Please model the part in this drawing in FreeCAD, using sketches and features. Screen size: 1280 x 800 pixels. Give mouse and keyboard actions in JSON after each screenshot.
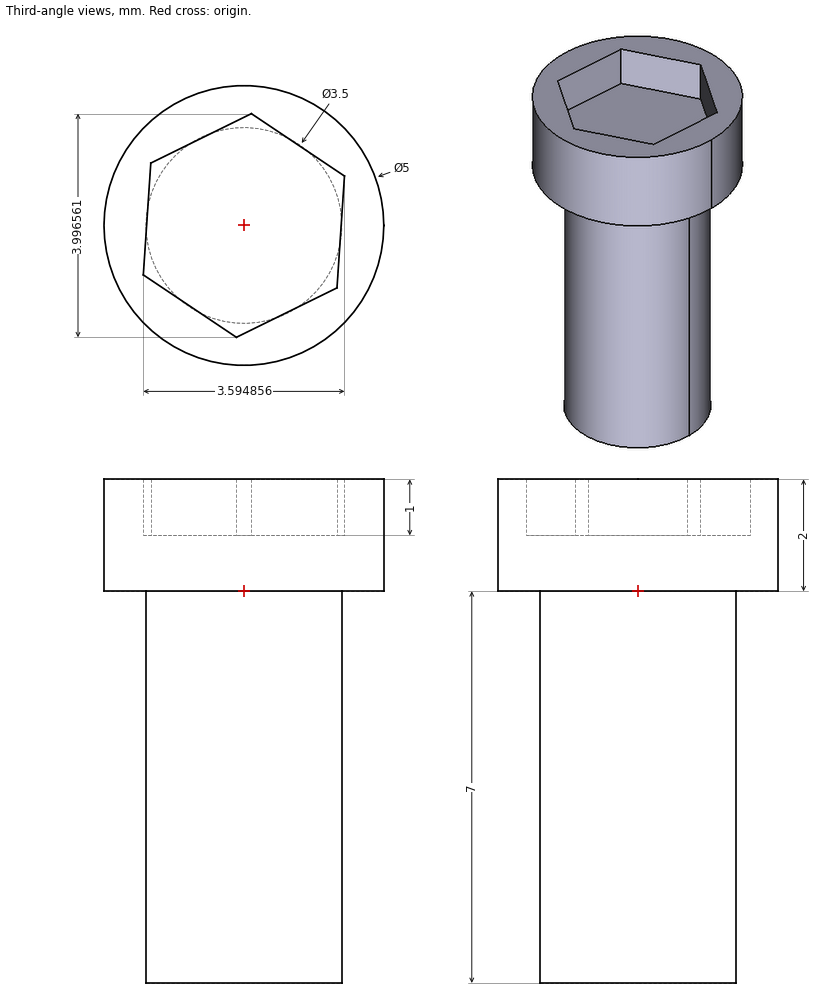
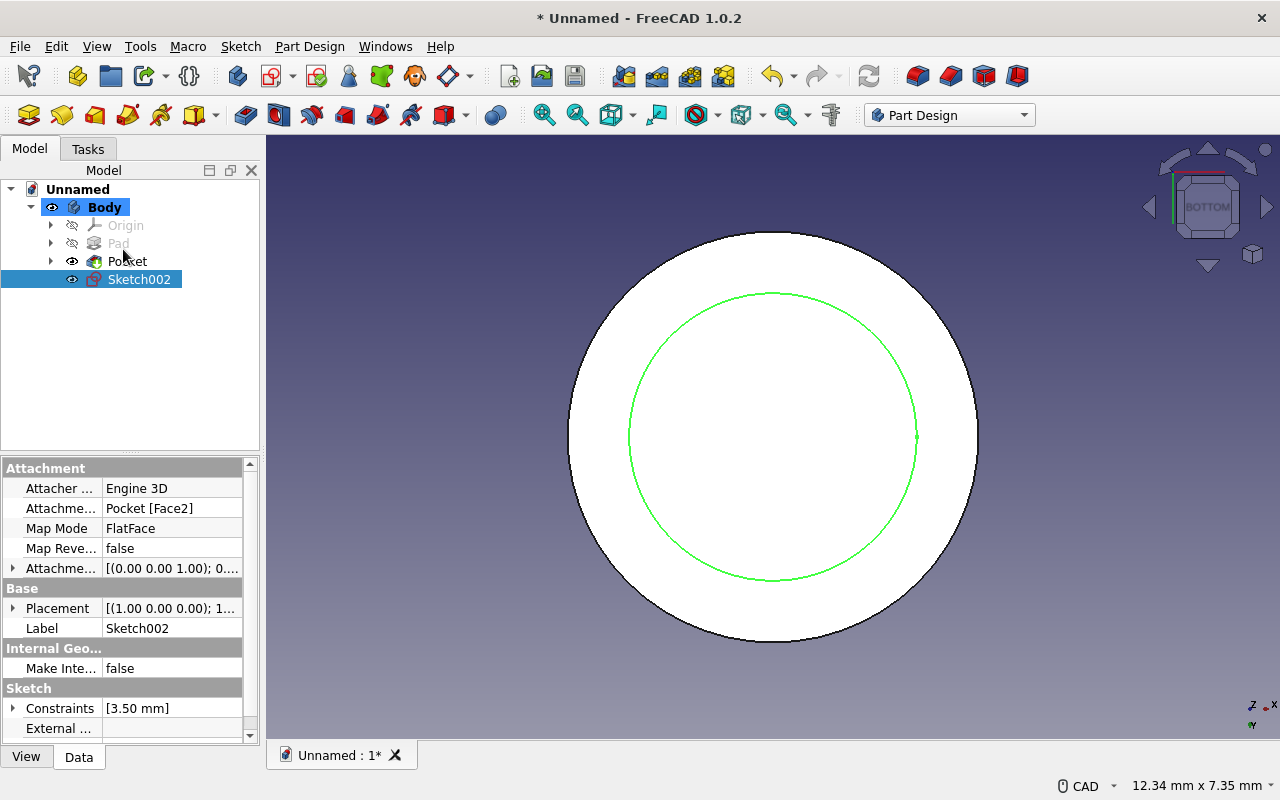
{"action": "left_click", "coordinate": [29, 116]}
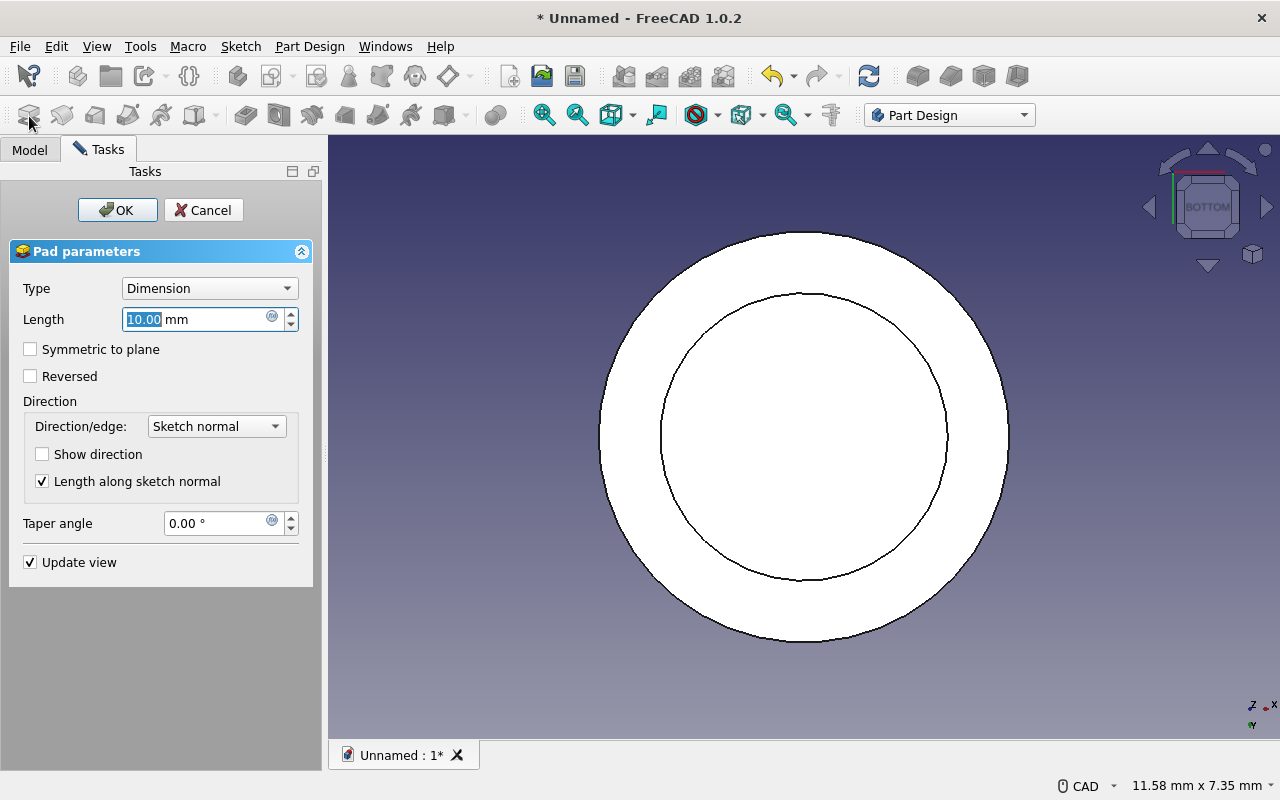
{"action": "type", "text": "7"}
{"action": "key", "text": "Tab"}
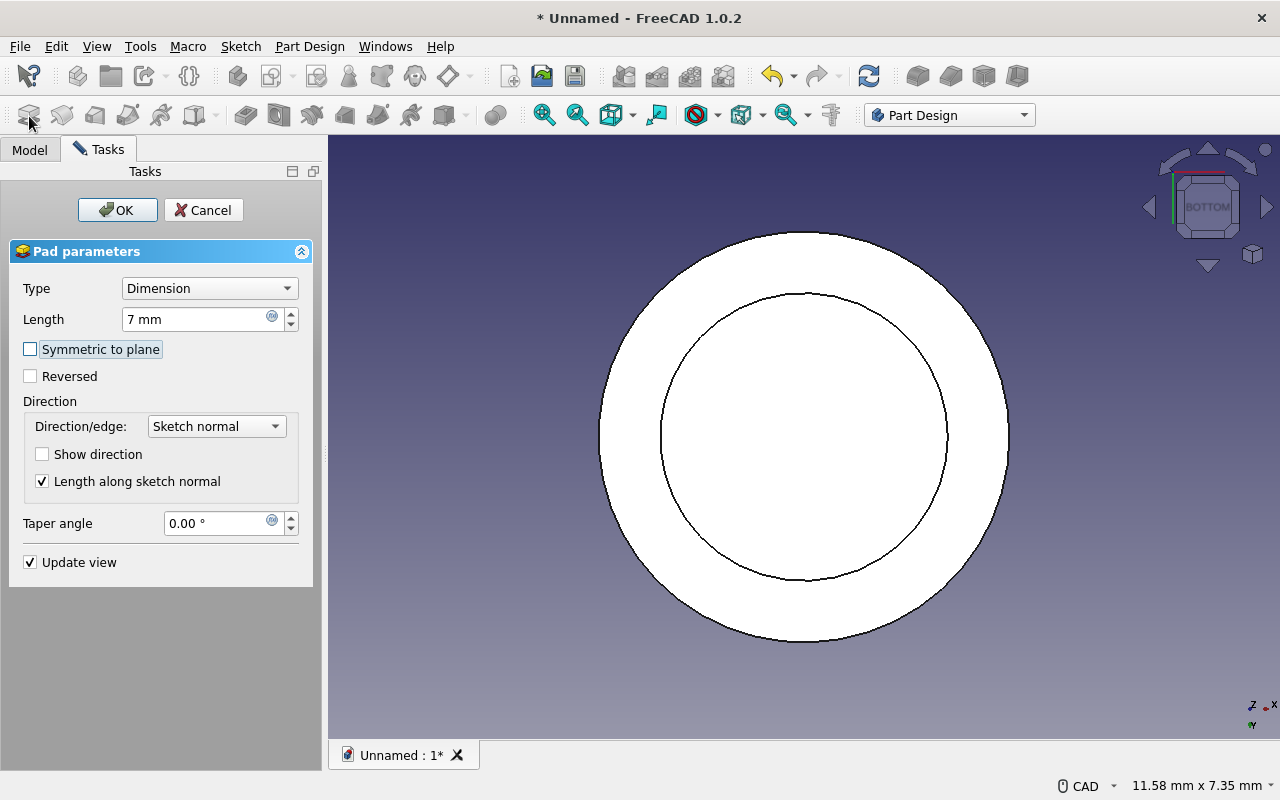
{"action": "left_click", "coordinate": [118, 210]}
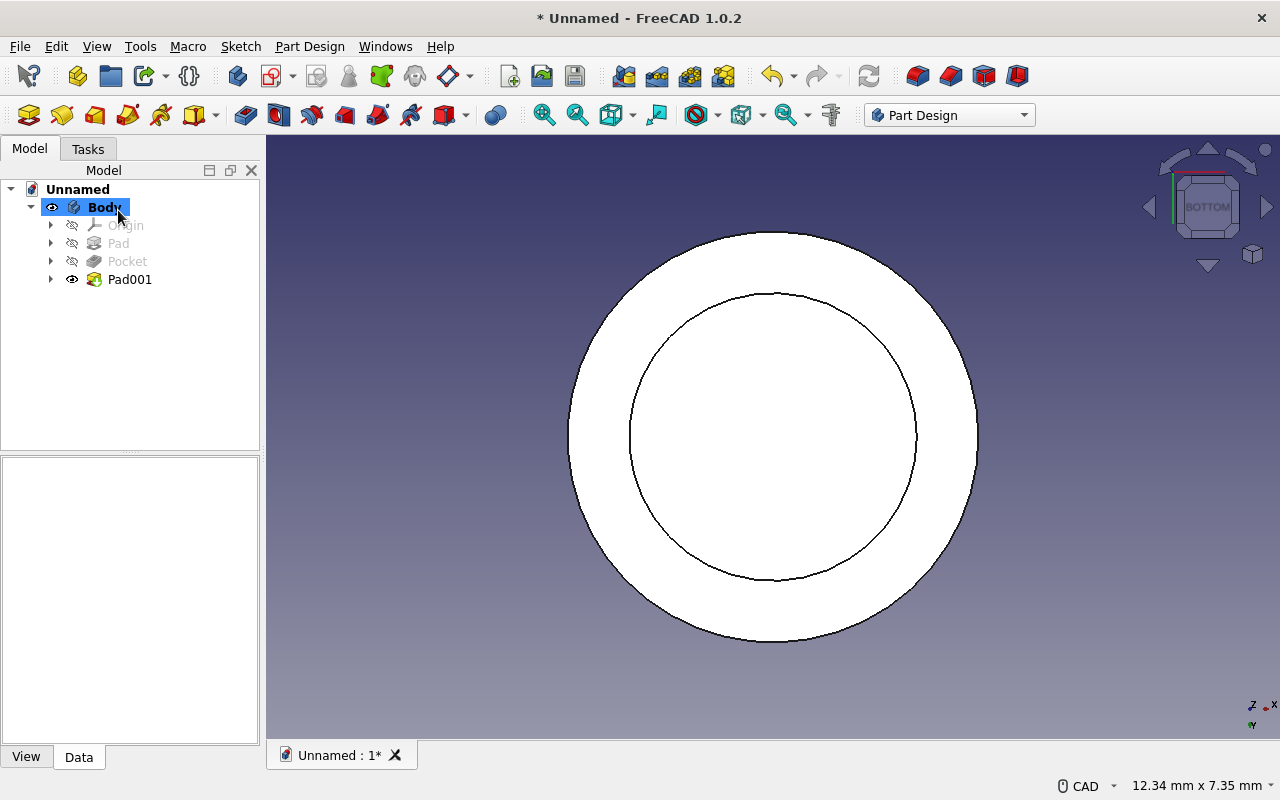
{"action": "key", "text": "0"}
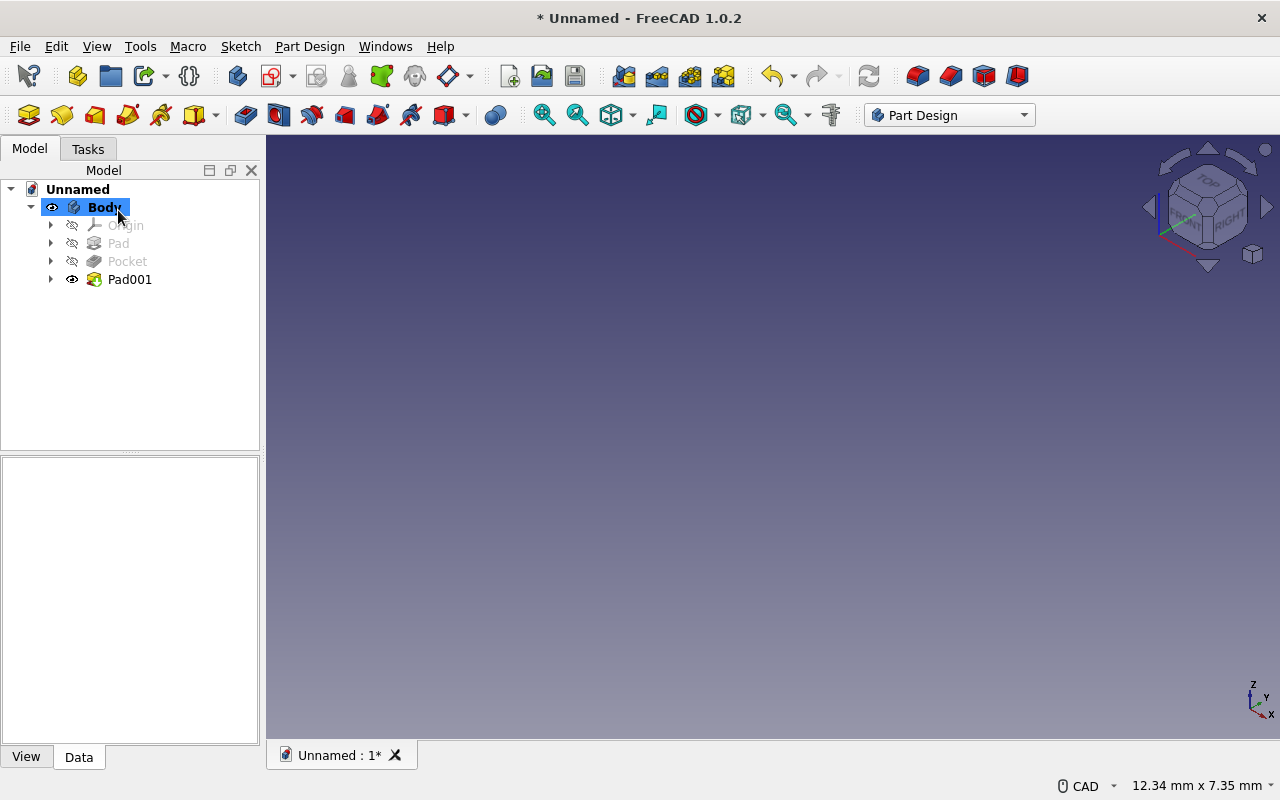
{"action": "left_click", "coordinate": [545, 116]}